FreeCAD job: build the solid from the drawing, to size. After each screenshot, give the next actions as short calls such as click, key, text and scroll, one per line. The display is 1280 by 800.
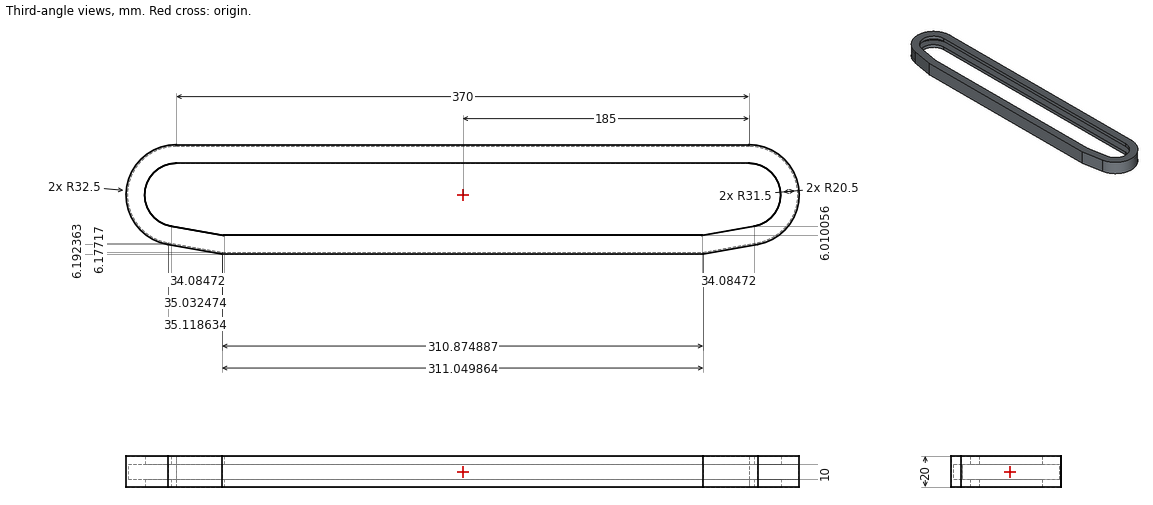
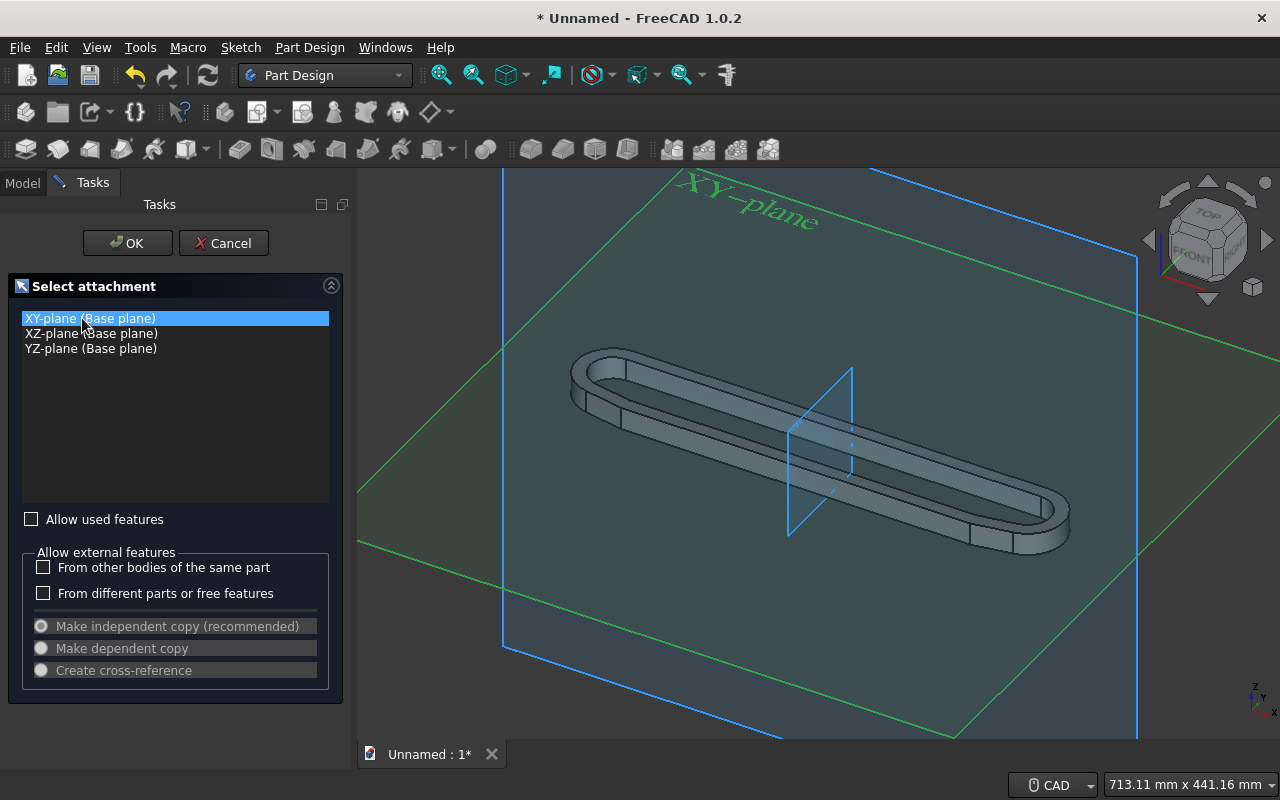
click(128, 243)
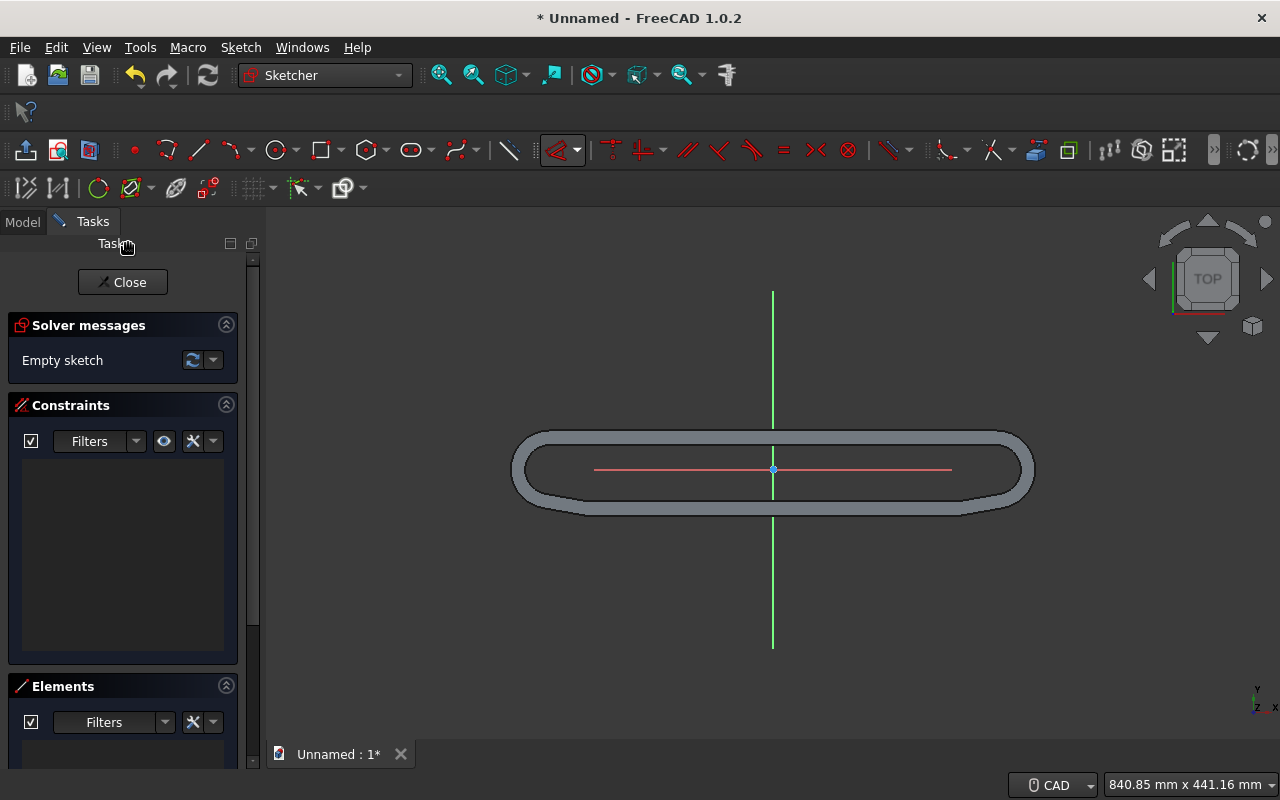
key(q)
key(s)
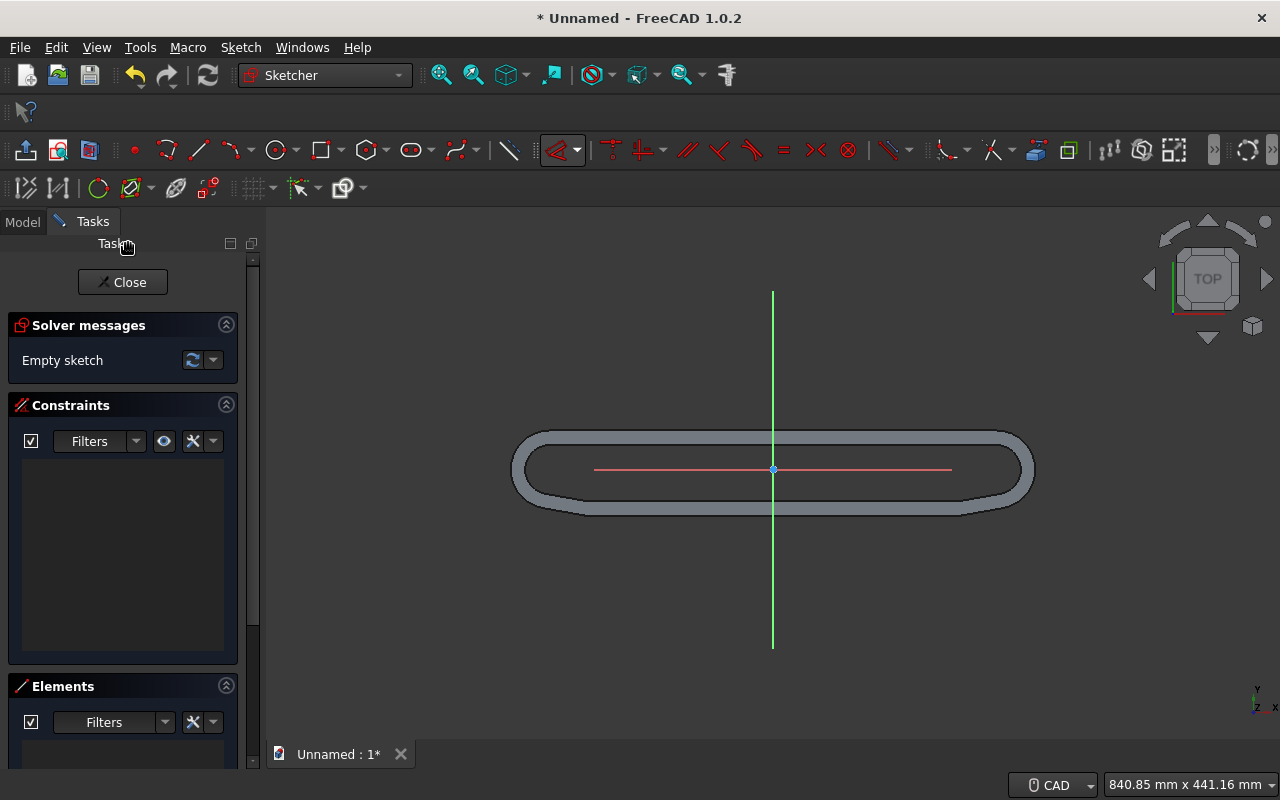
key(g)
key(l)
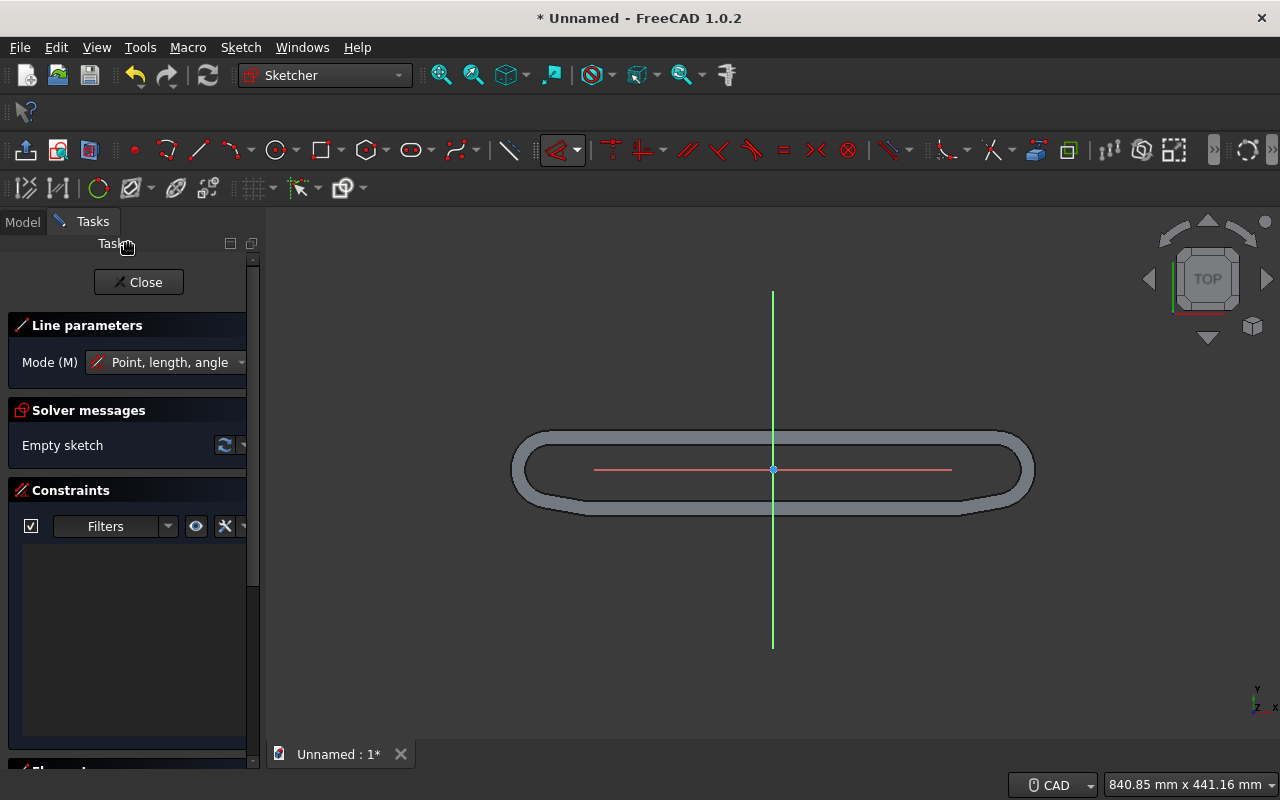
click(996, 432)
click(550, 432)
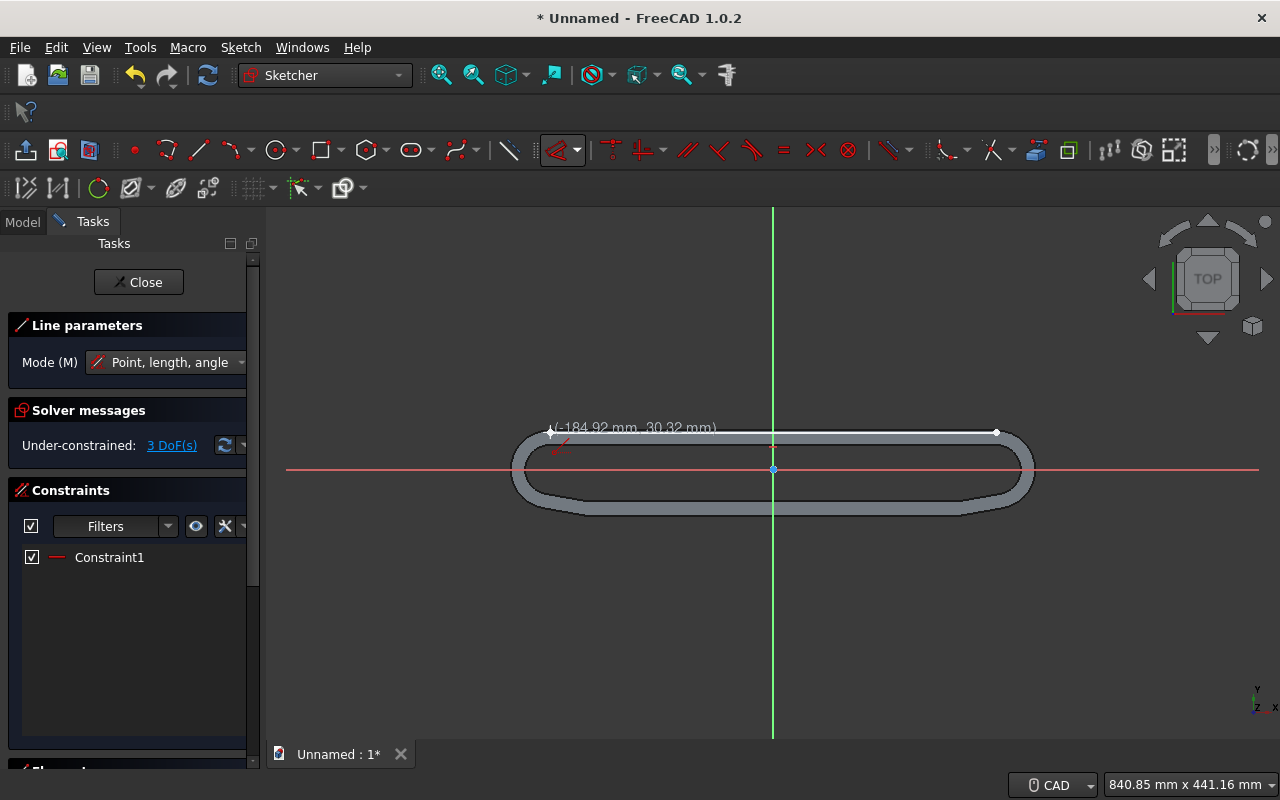
click(168, 150)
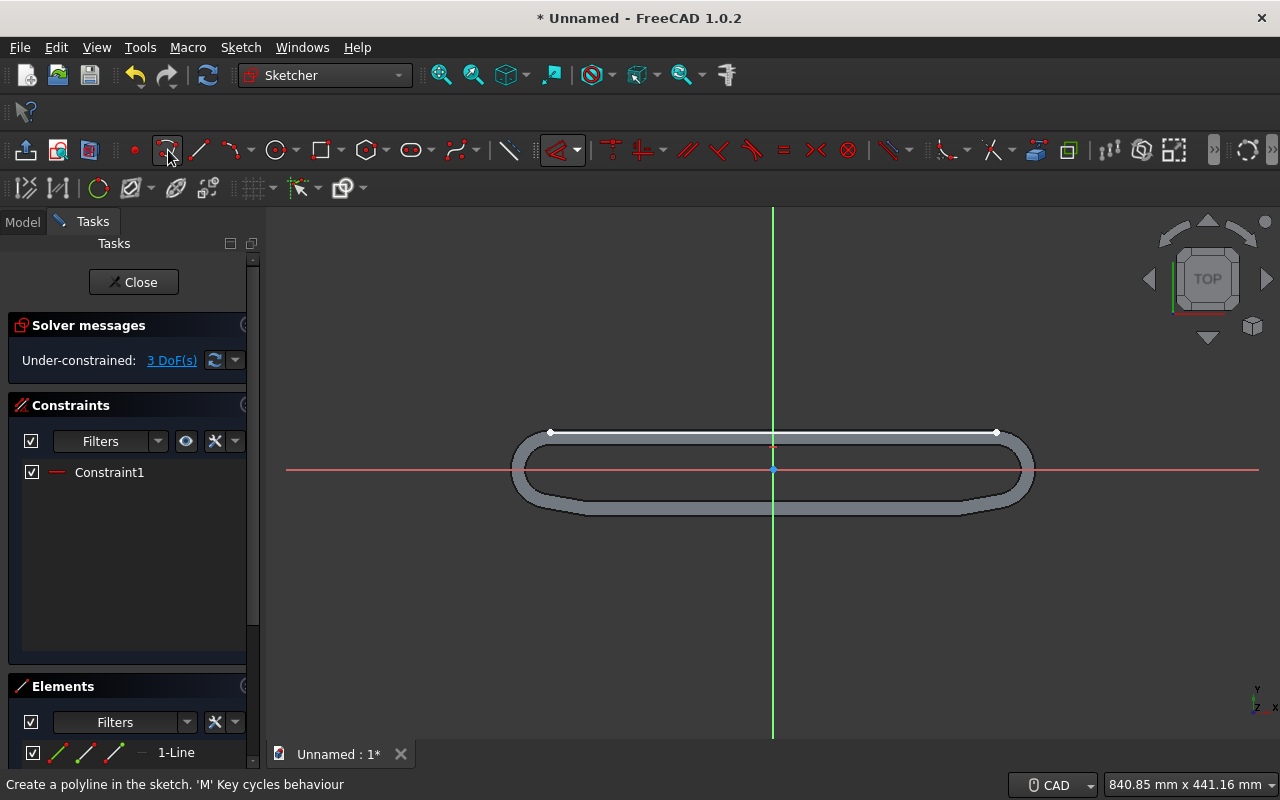
click(543, 507)
click(586, 514)
click(960, 514)
click(1003, 507)
right_click(1003, 507)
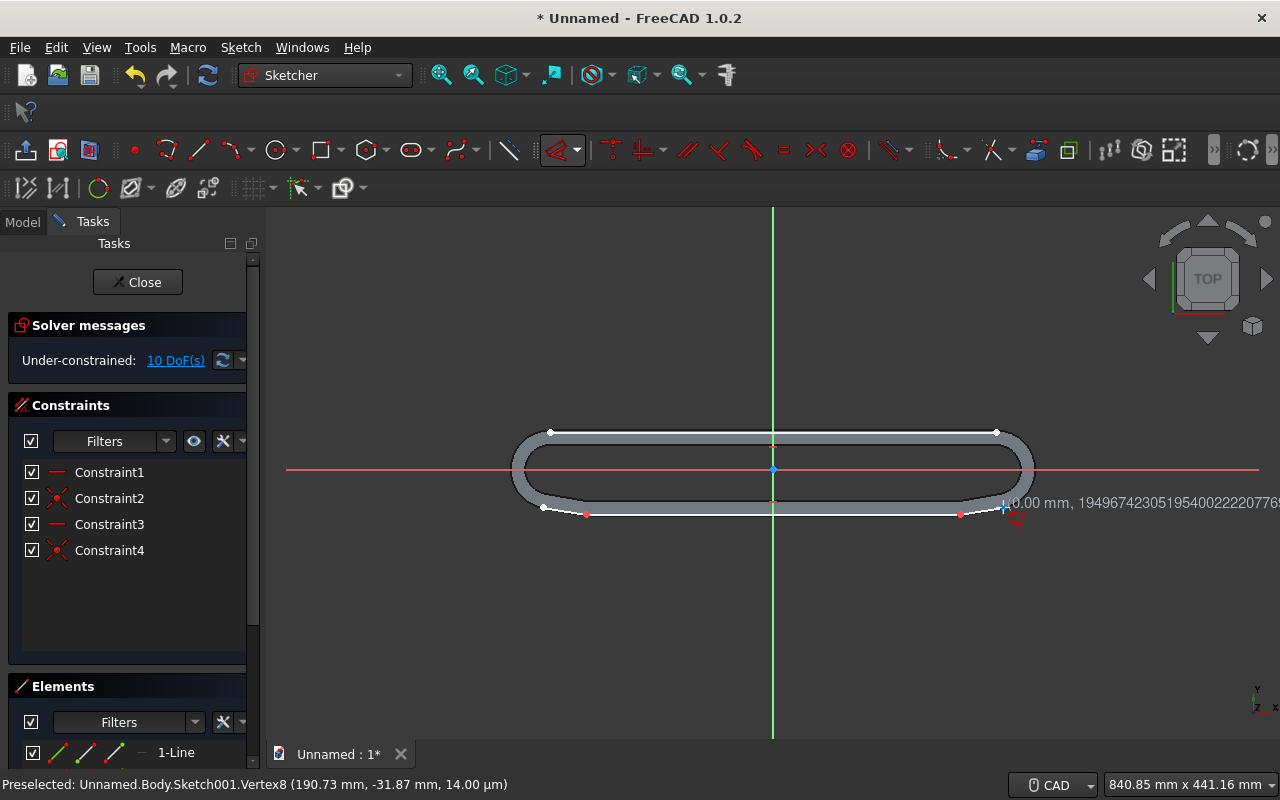
key(g)
key(3)
key(a)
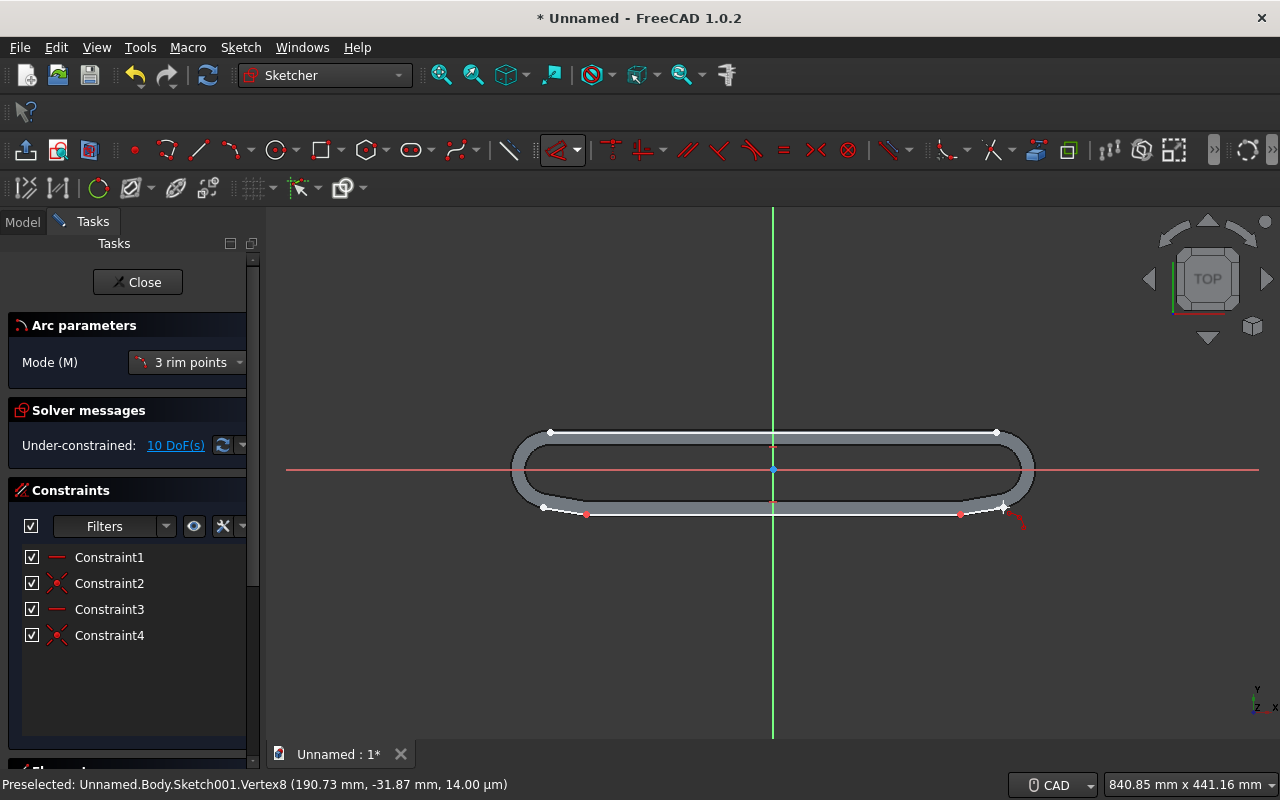
click(550, 433)
click(543, 508)
click(515, 455)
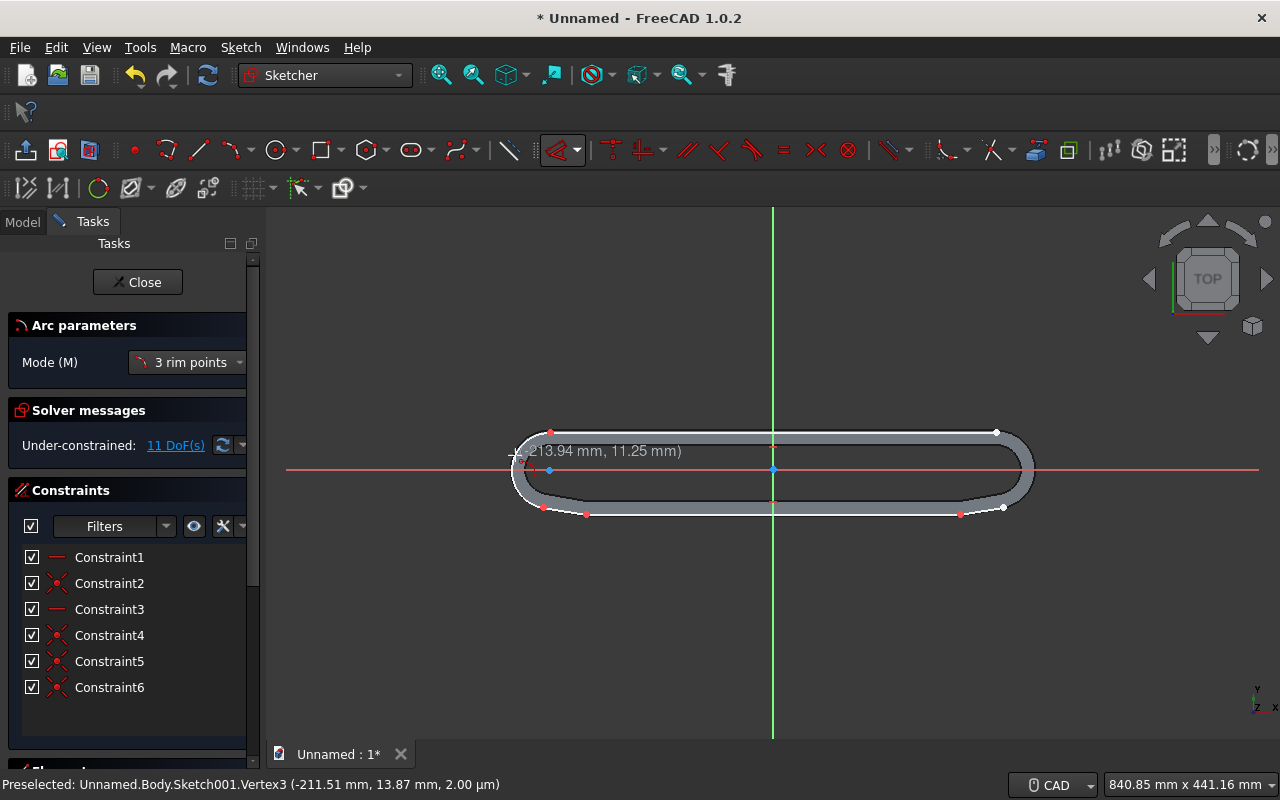
click(1003, 508)
click(996, 433)
click(1031, 455)
key(Escape)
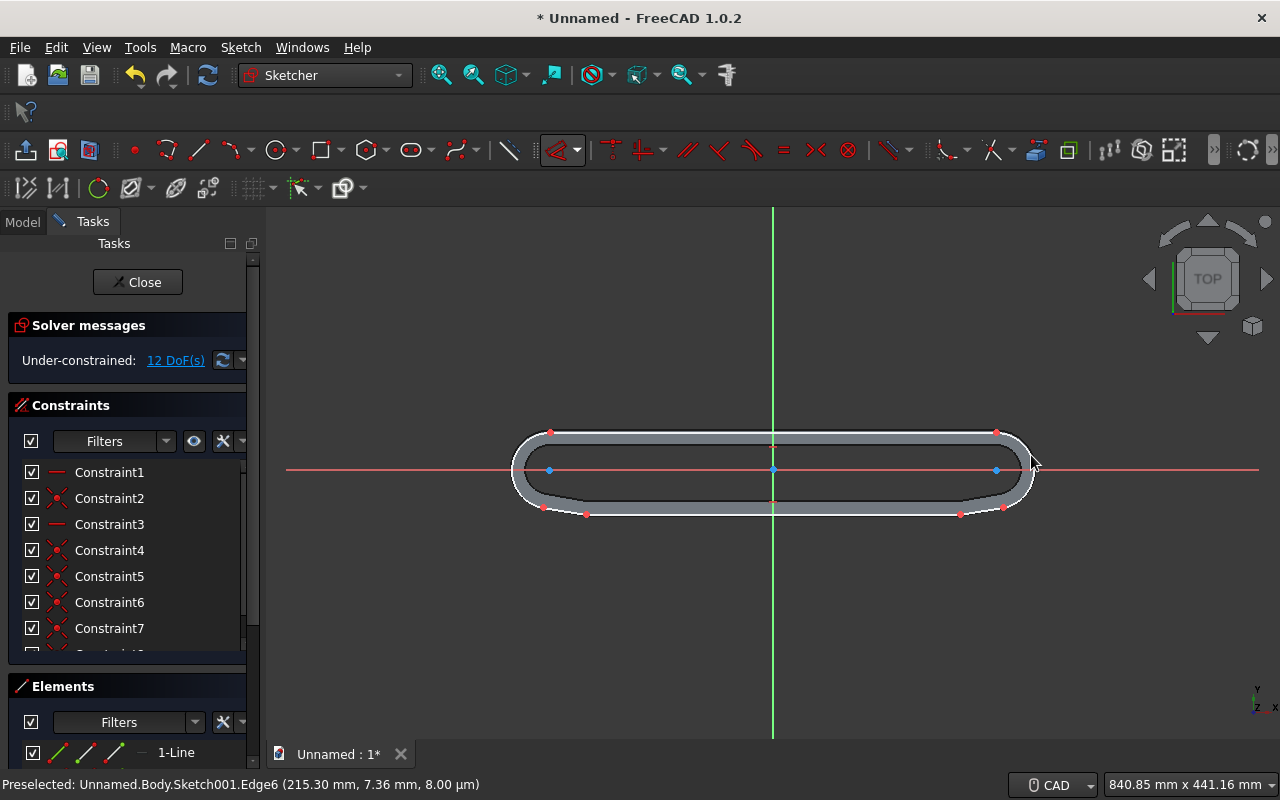
click(862, 433)